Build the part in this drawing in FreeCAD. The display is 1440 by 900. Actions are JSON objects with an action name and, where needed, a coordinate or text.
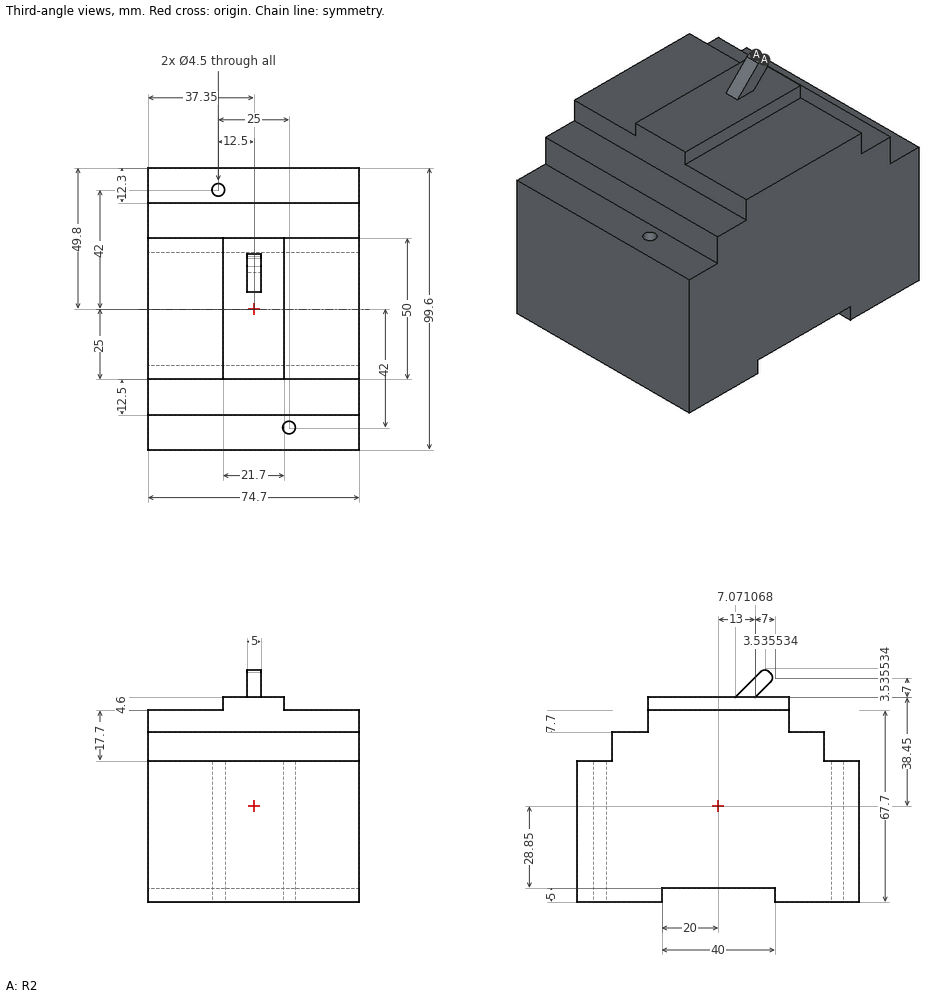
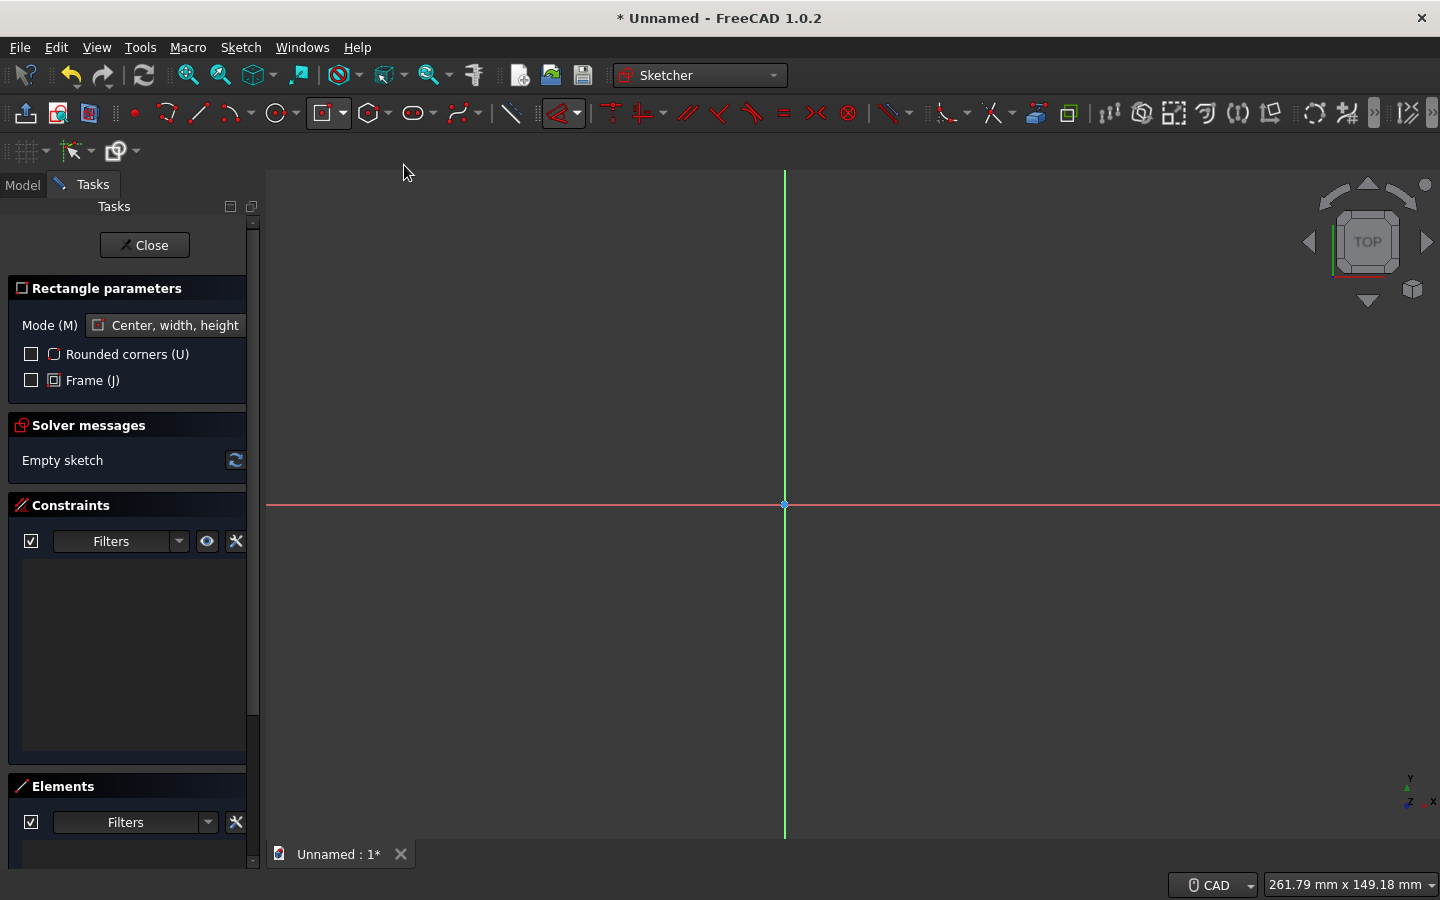
{"action": "left_click", "coordinate": [785, 505]}
{"action": "left_click", "coordinate": [952, 282]}
{"action": "key", "text": "Escape"}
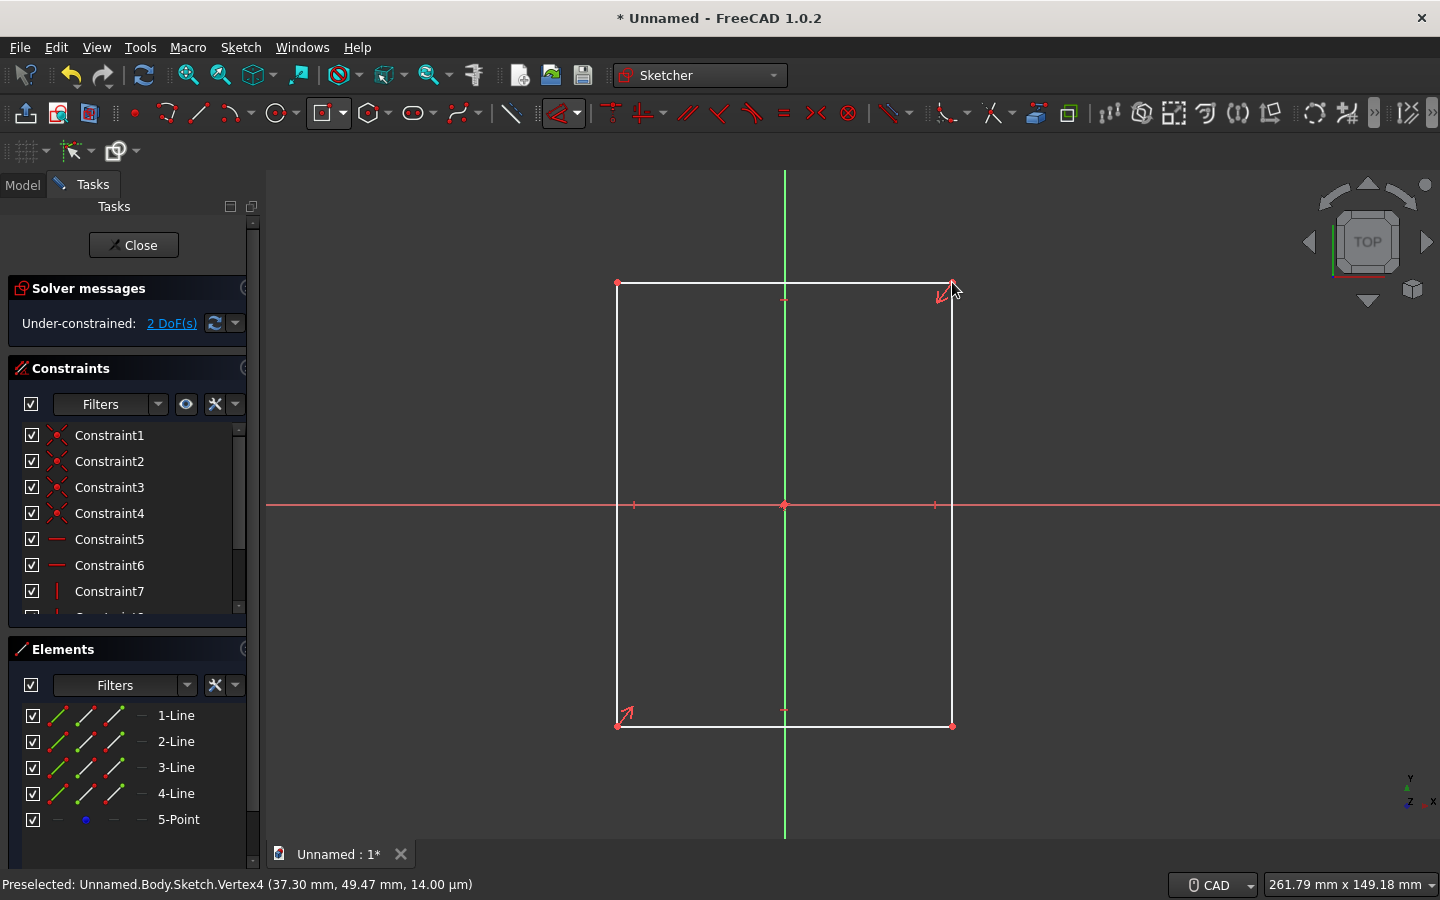
{"action": "left_click", "coordinate": [558, 114]}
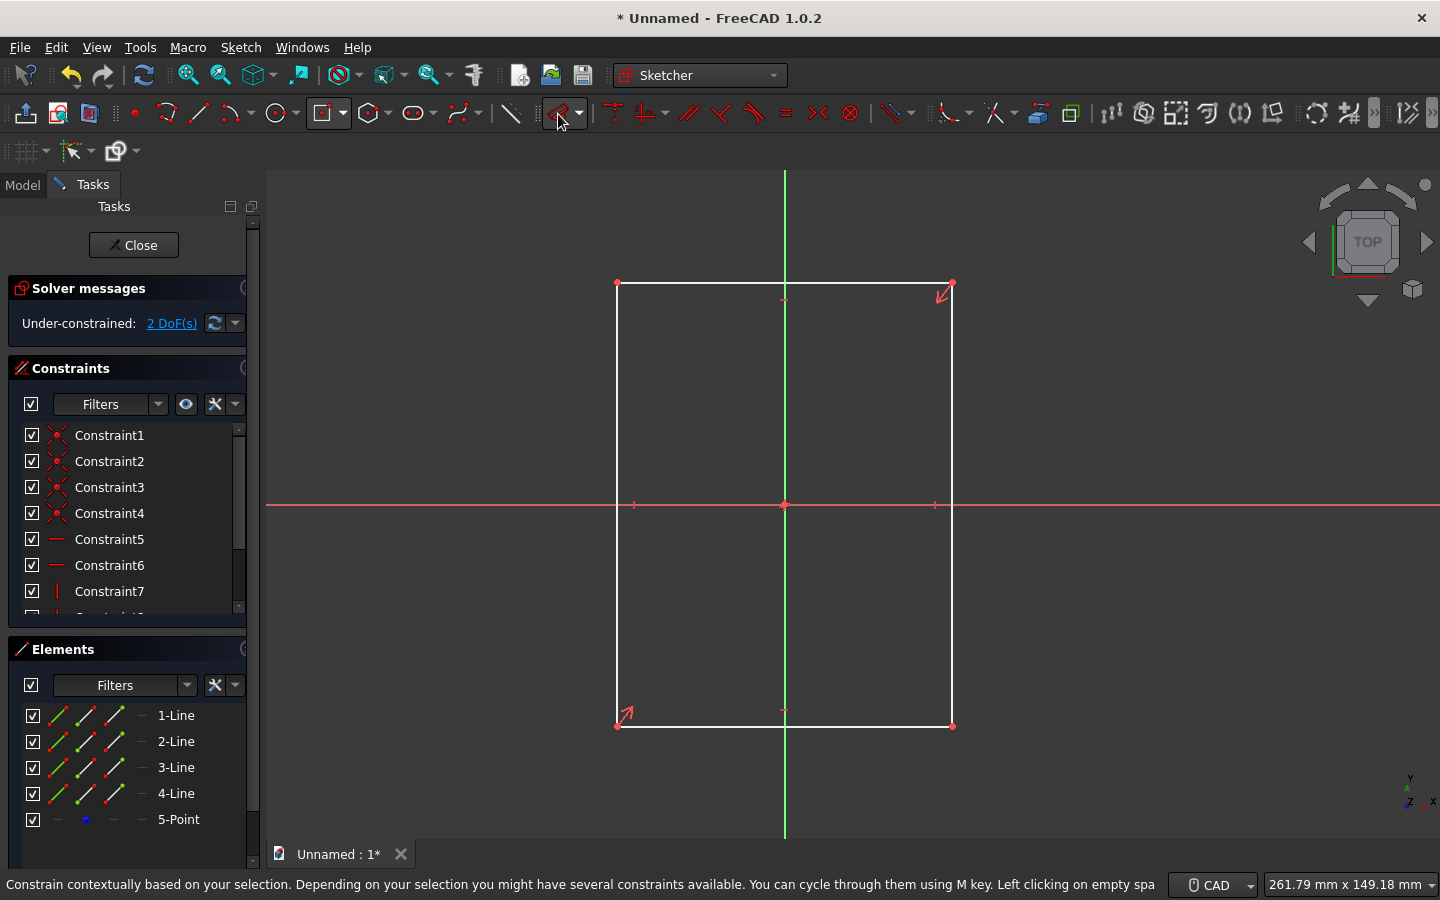
{"action": "left_click", "coordinate": [718, 727]}
{"action": "left_click", "coordinate": [708, 761]}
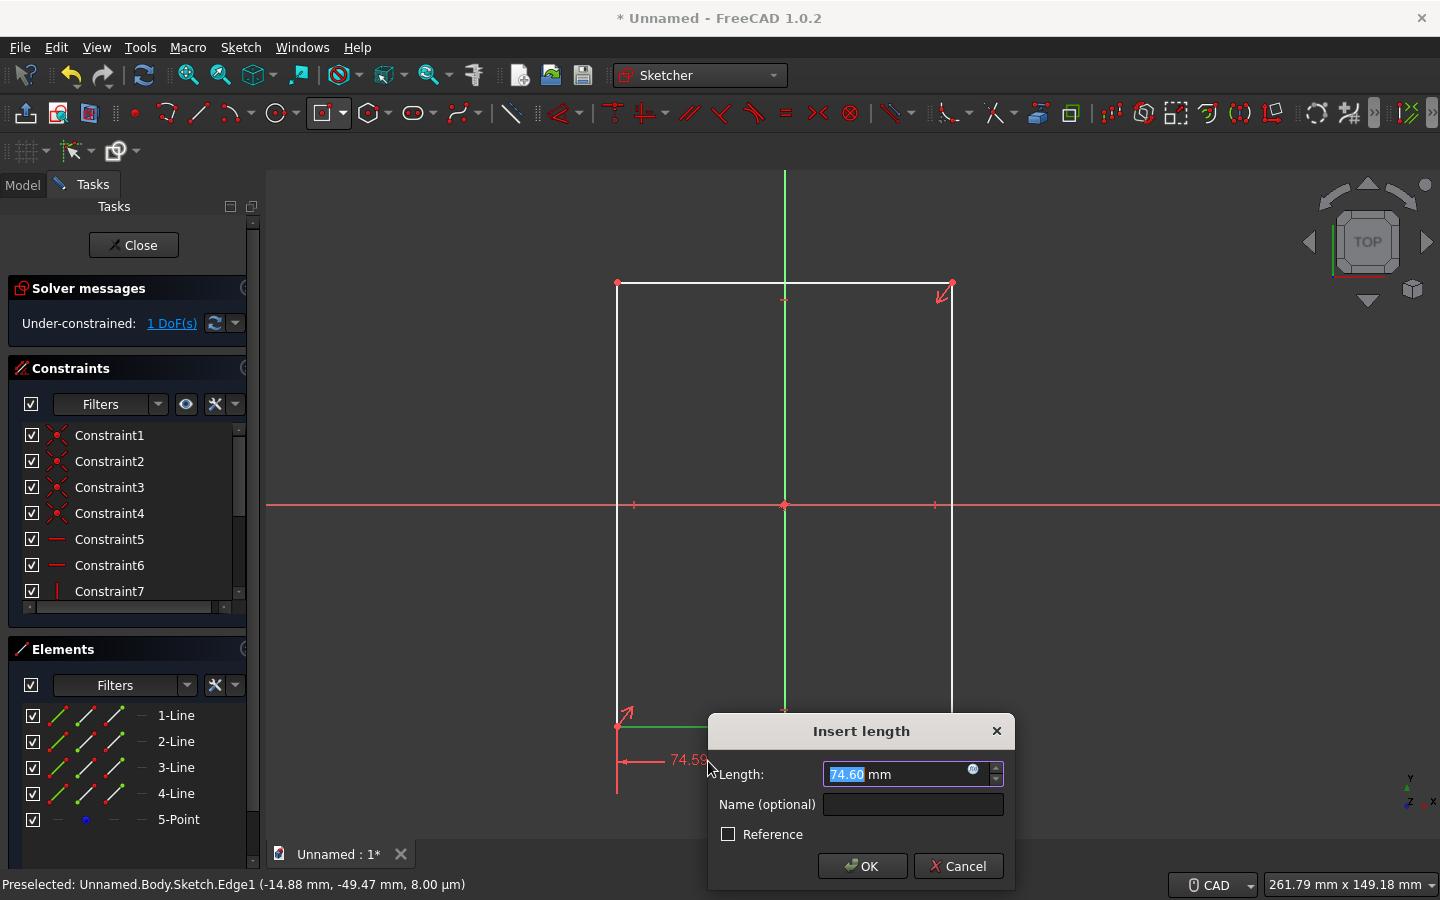
{"action": "type", "text": "74.7"}
{"action": "key", "text": "Return"}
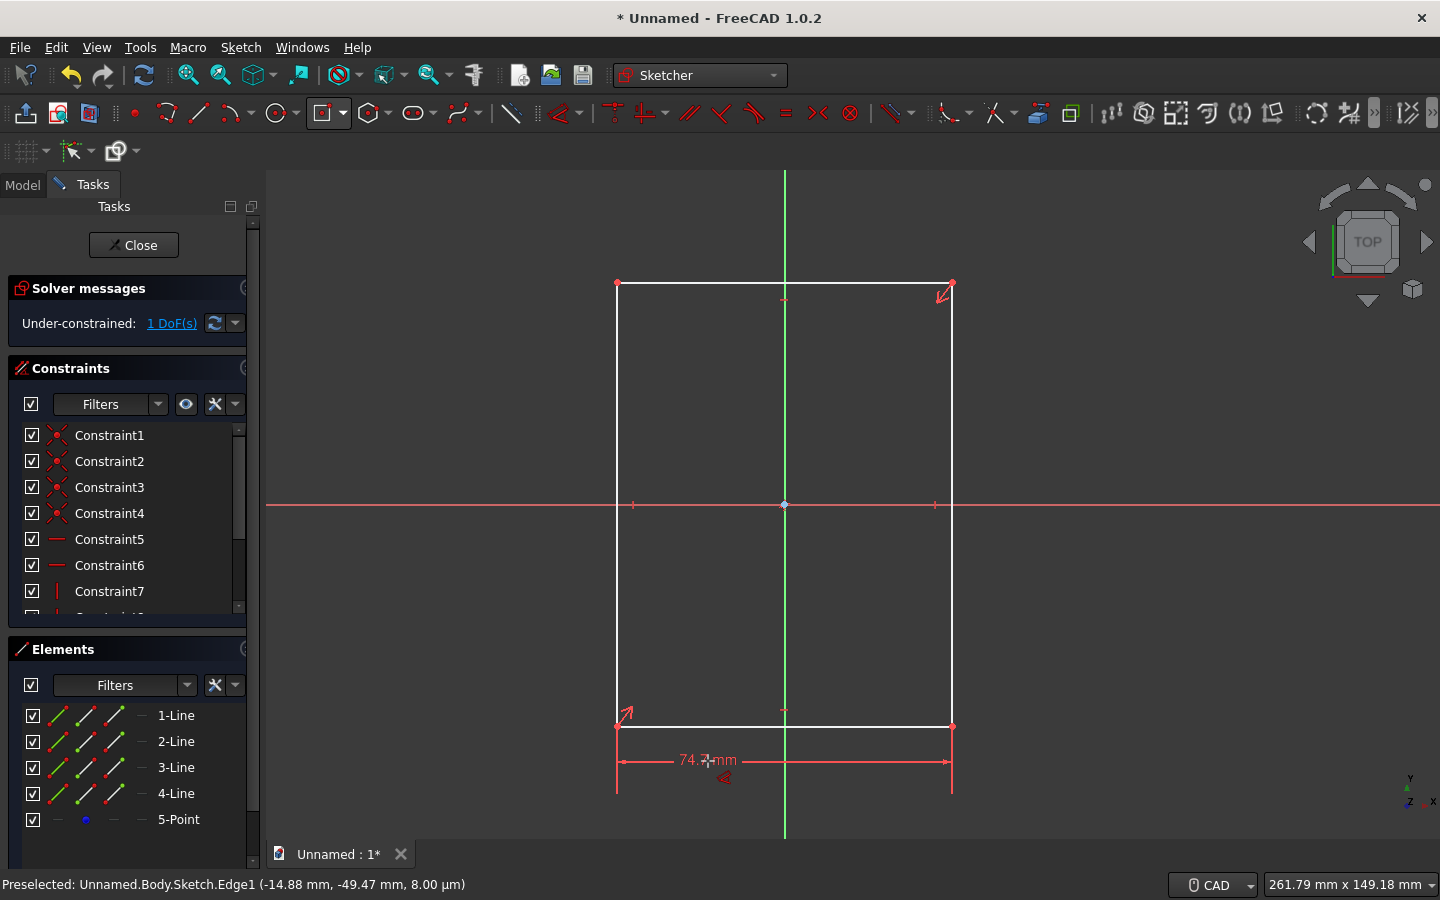
{"action": "left_click", "coordinate": [952, 594]}
{"action": "left_click", "coordinate": [986, 403]}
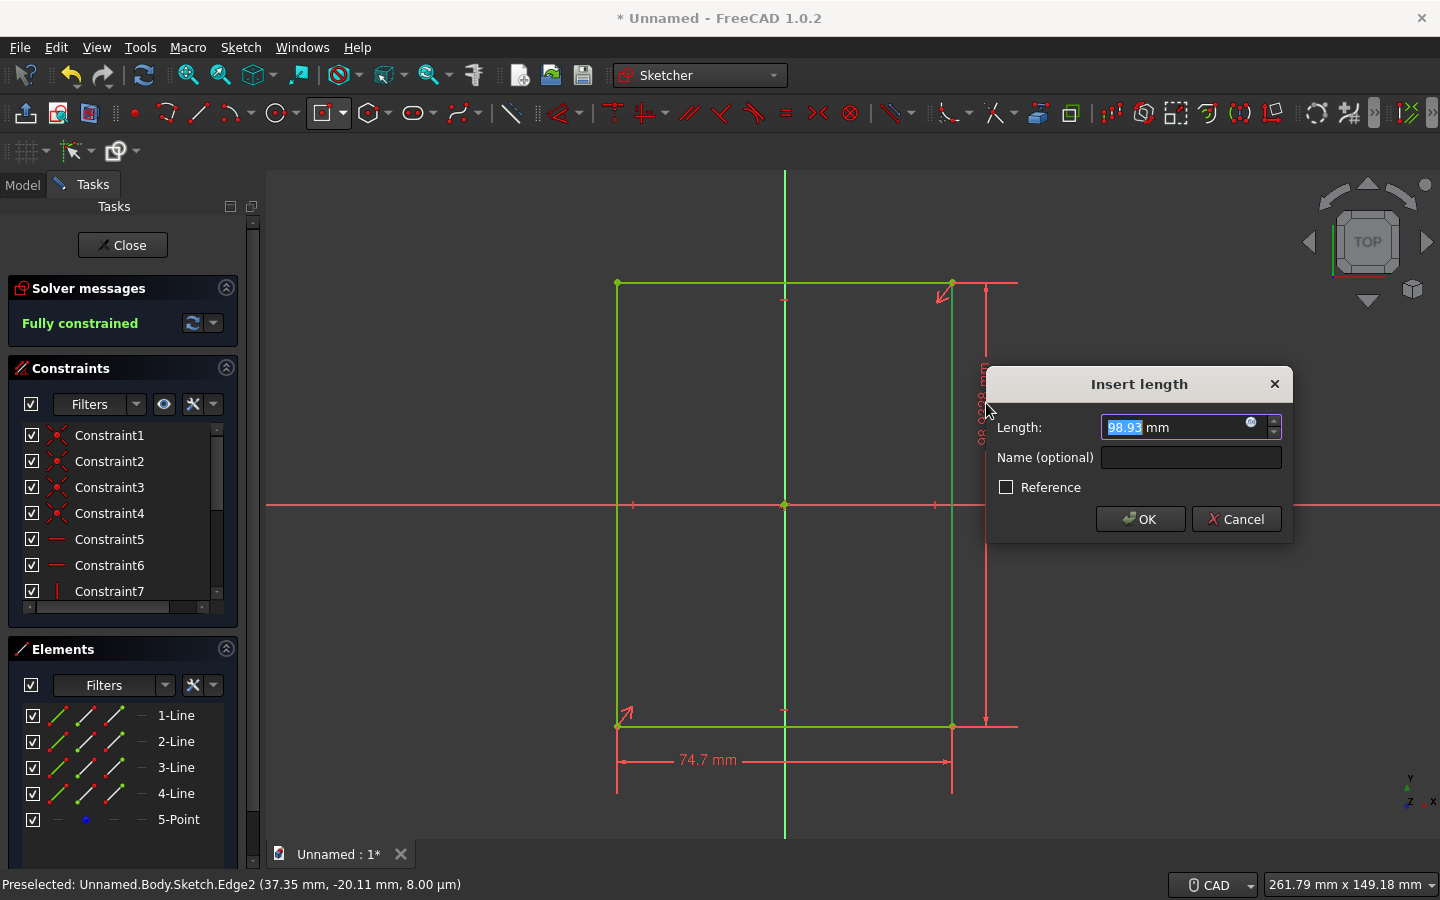
{"action": "type", "text": "99.6"}
{"action": "key", "text": "Return"}
{"action": "key", "text": "Escape"}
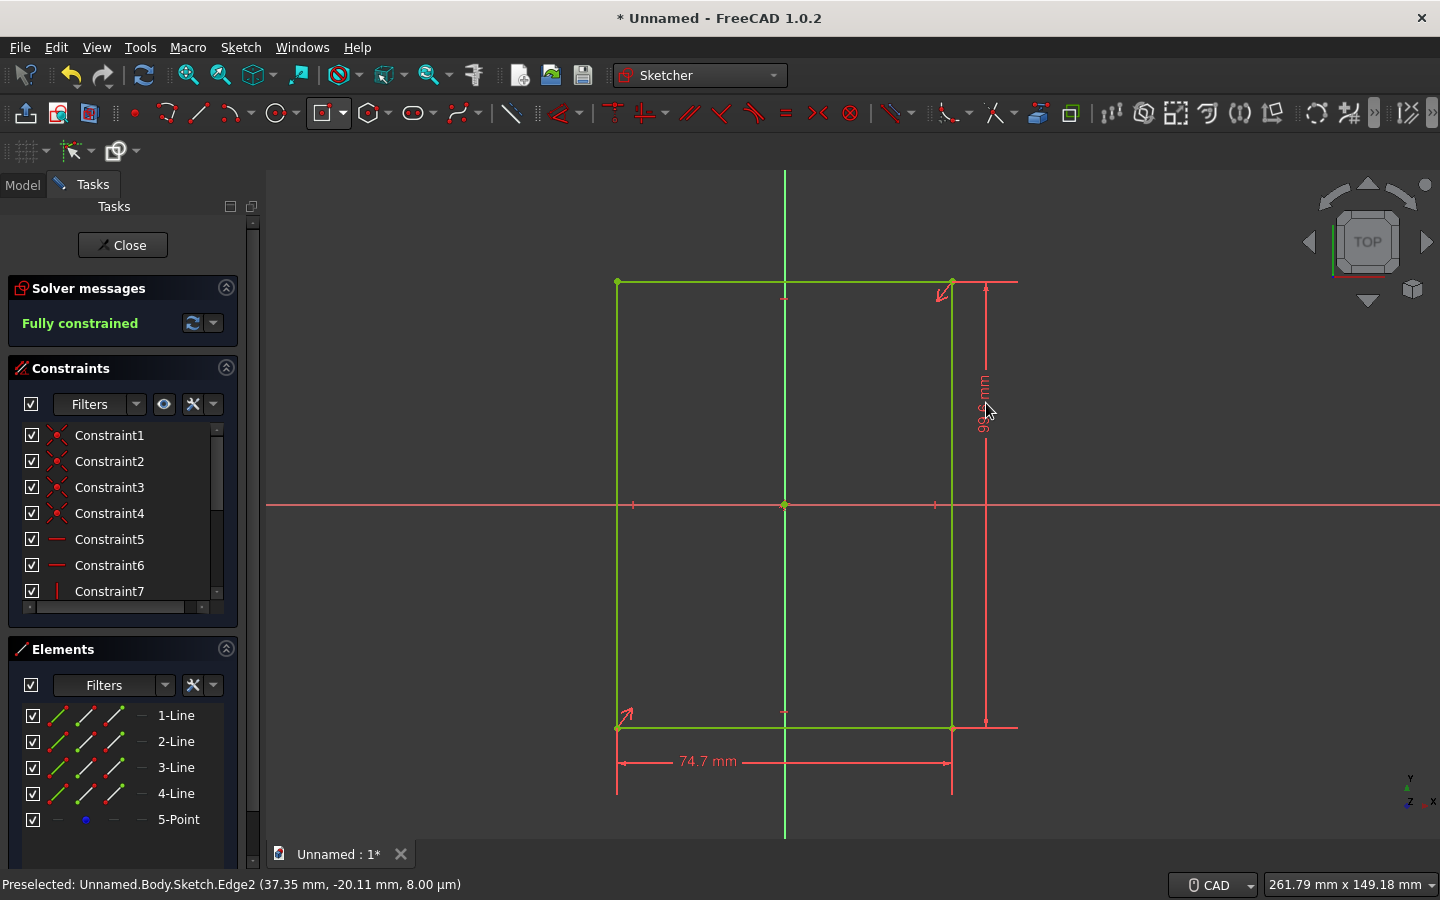
{"action": "left_click", "coordinate": [123, 245]}